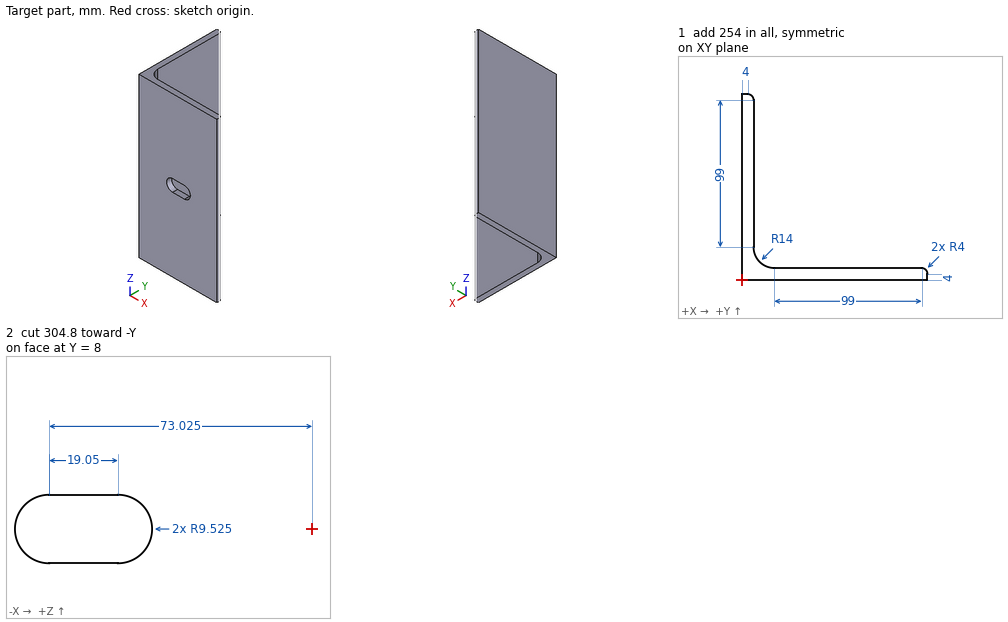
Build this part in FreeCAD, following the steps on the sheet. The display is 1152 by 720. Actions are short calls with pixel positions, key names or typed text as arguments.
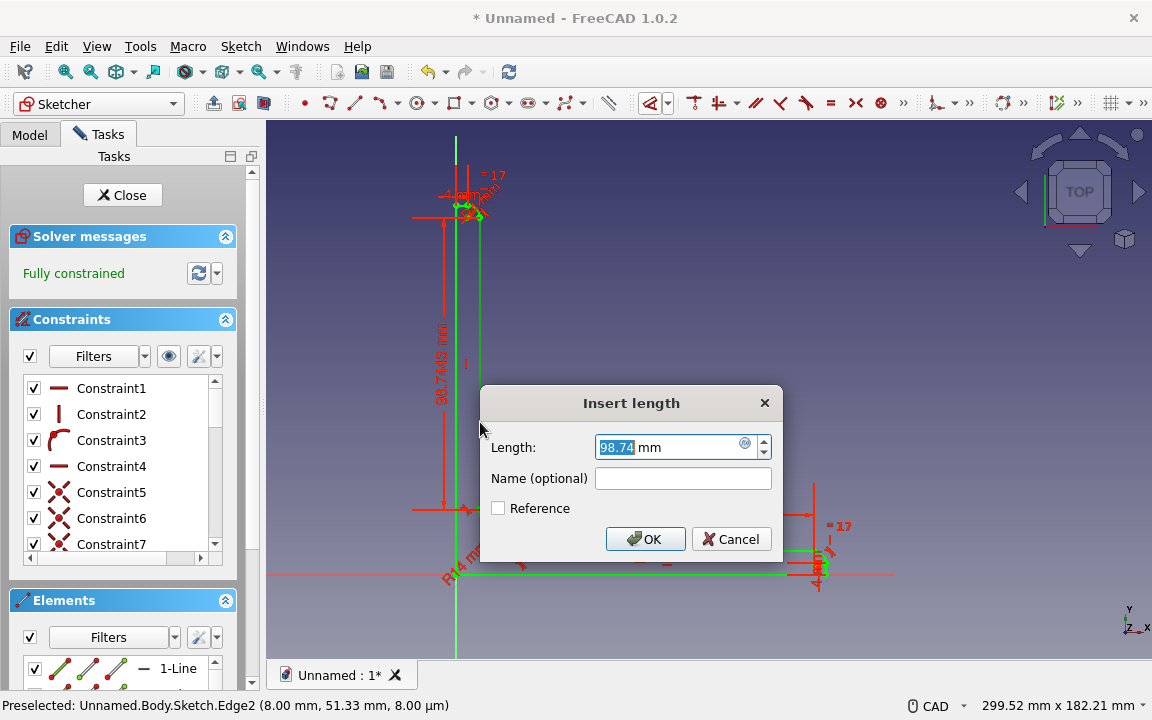
text(99)
key(Return)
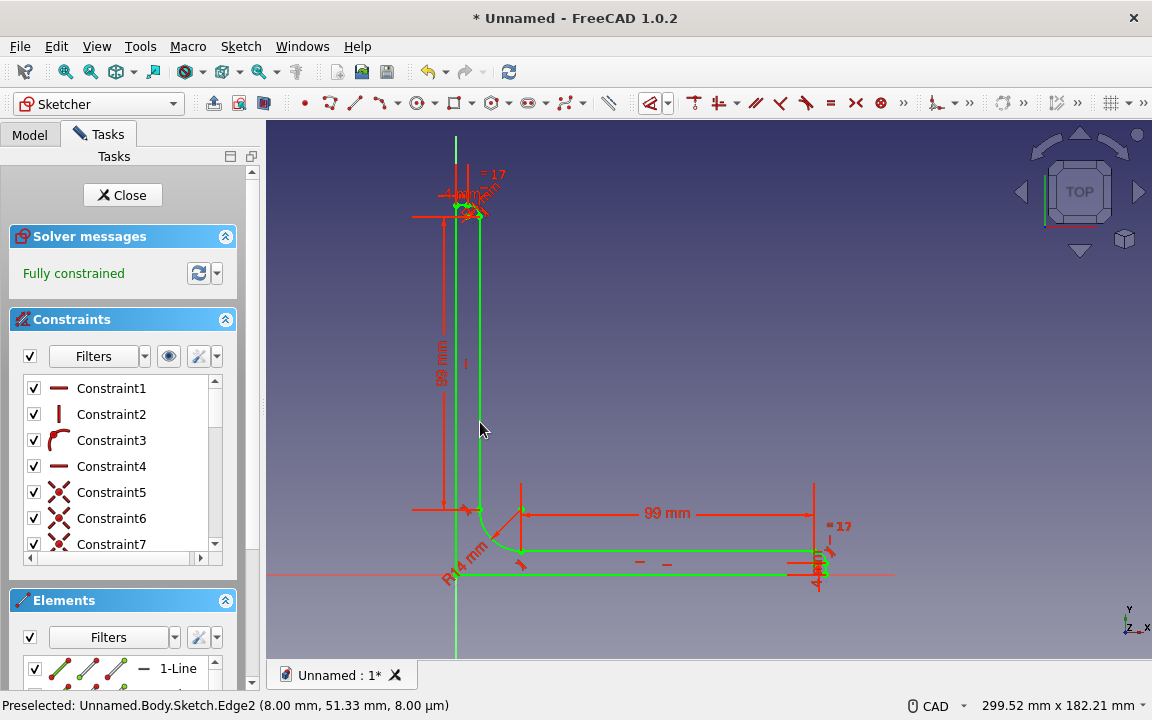
click(123, 195)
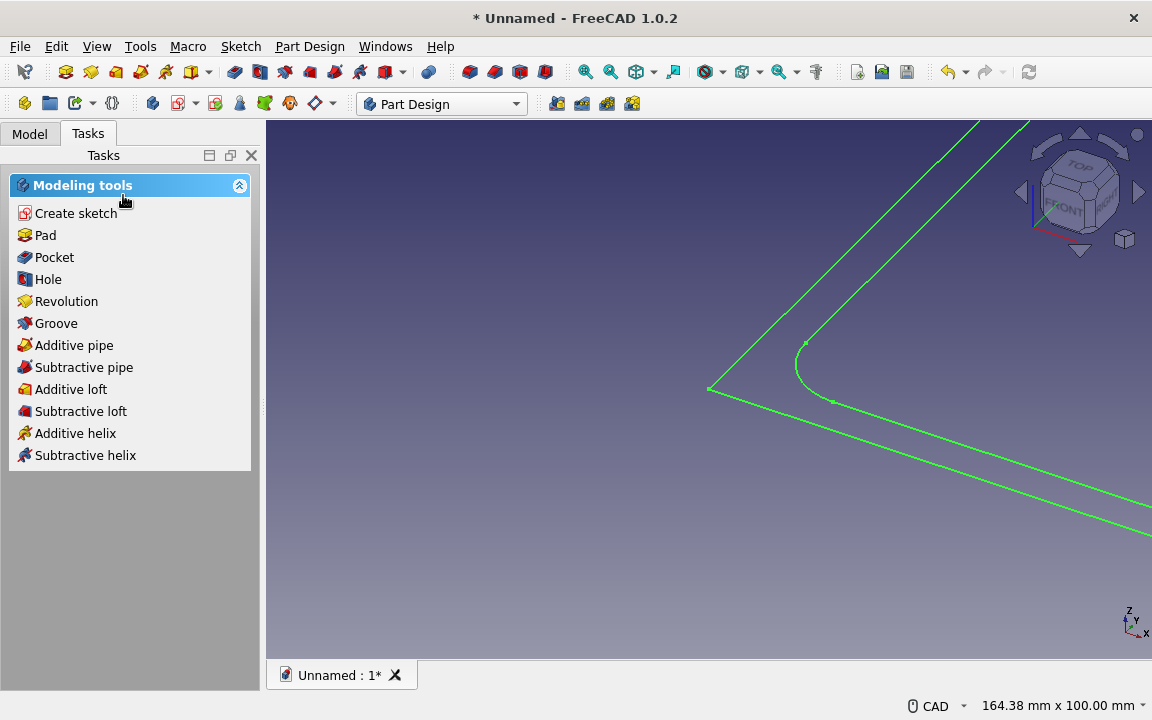
click(66, 72)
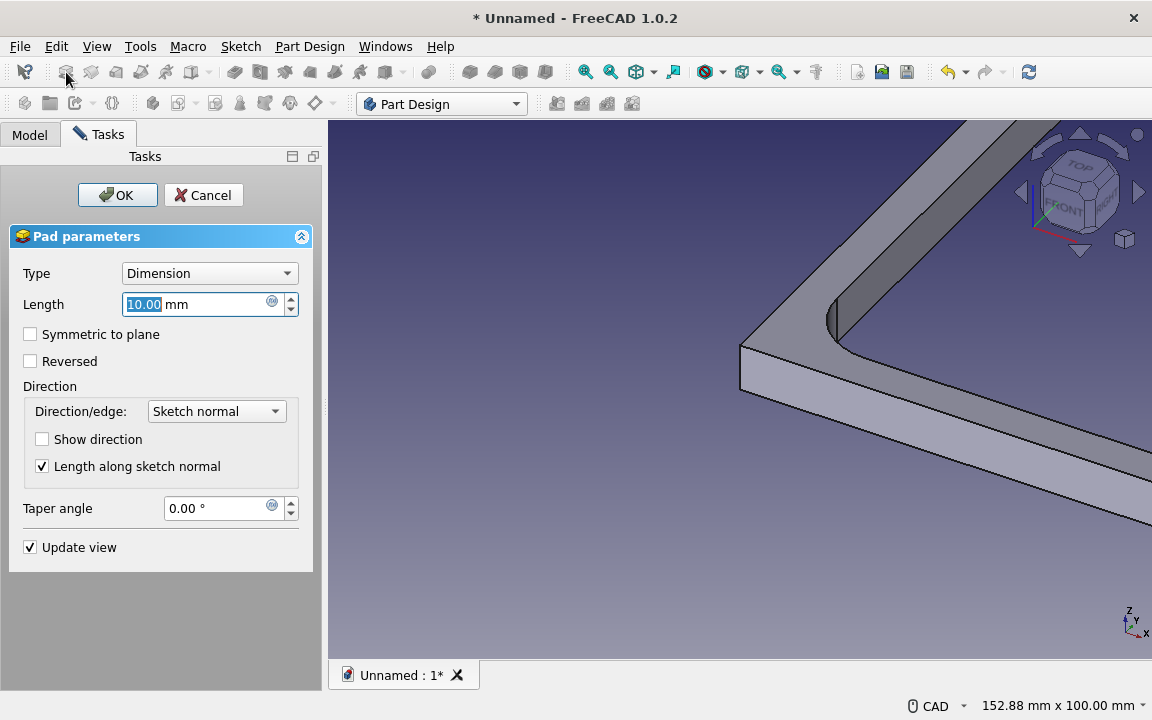
text(254)
key(Tab)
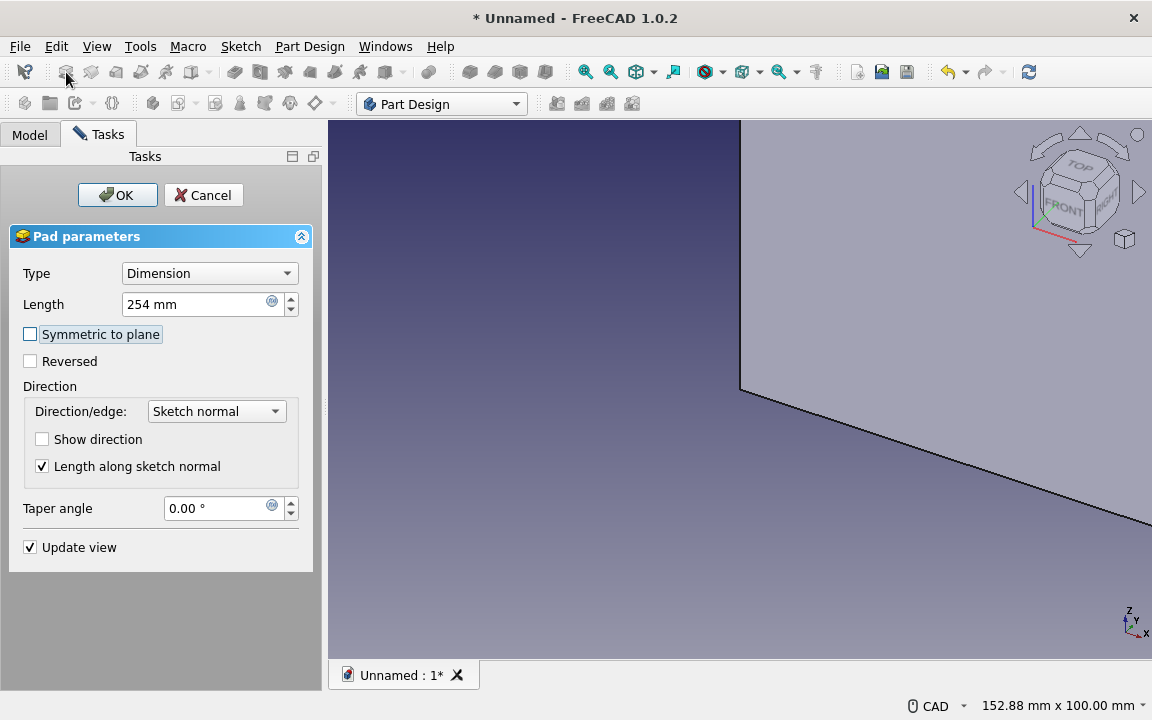
click(31, 334)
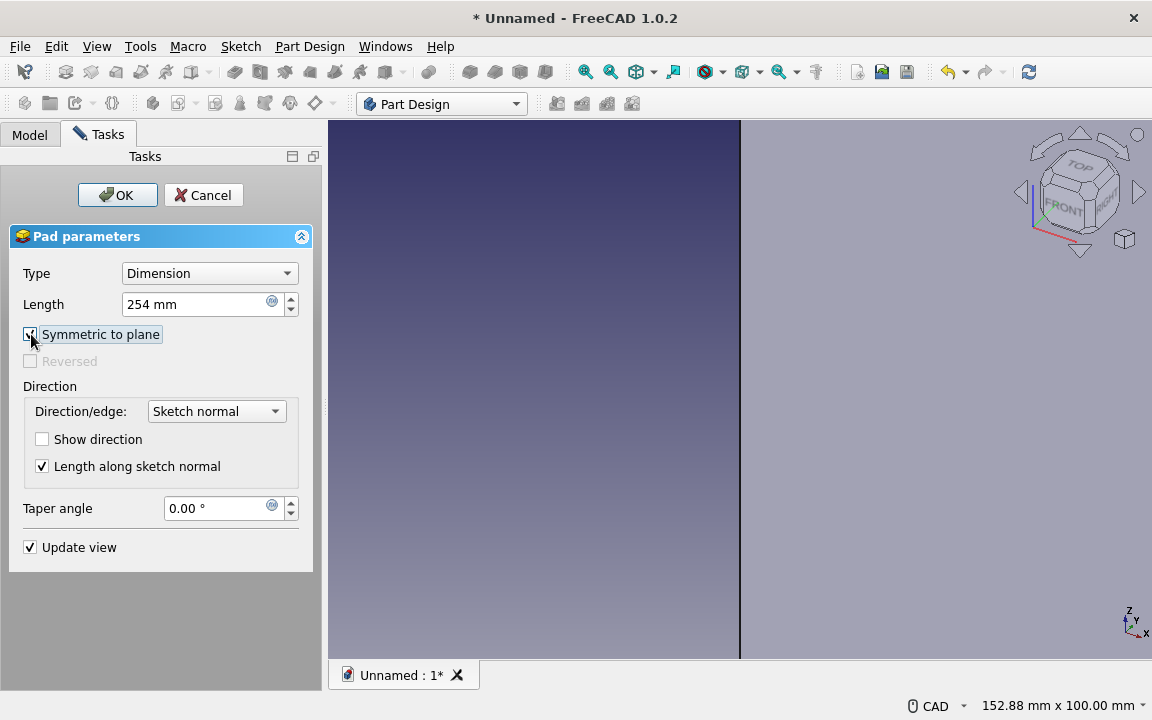
click(118, 195)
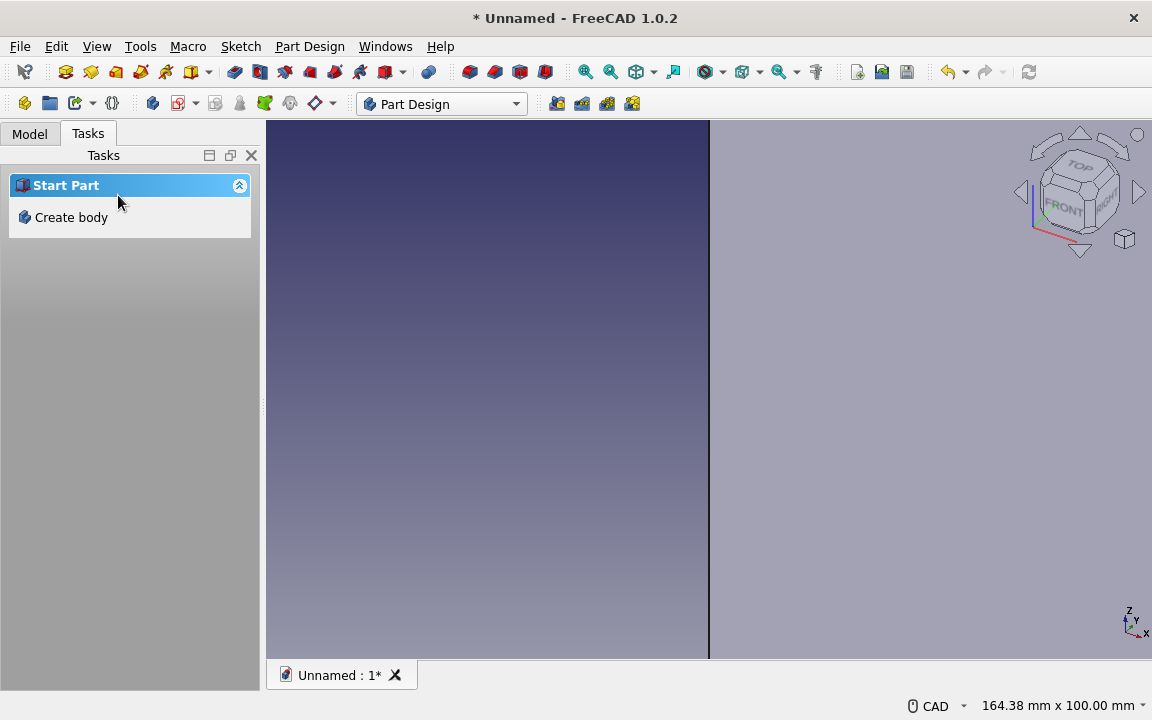
click(586, 72)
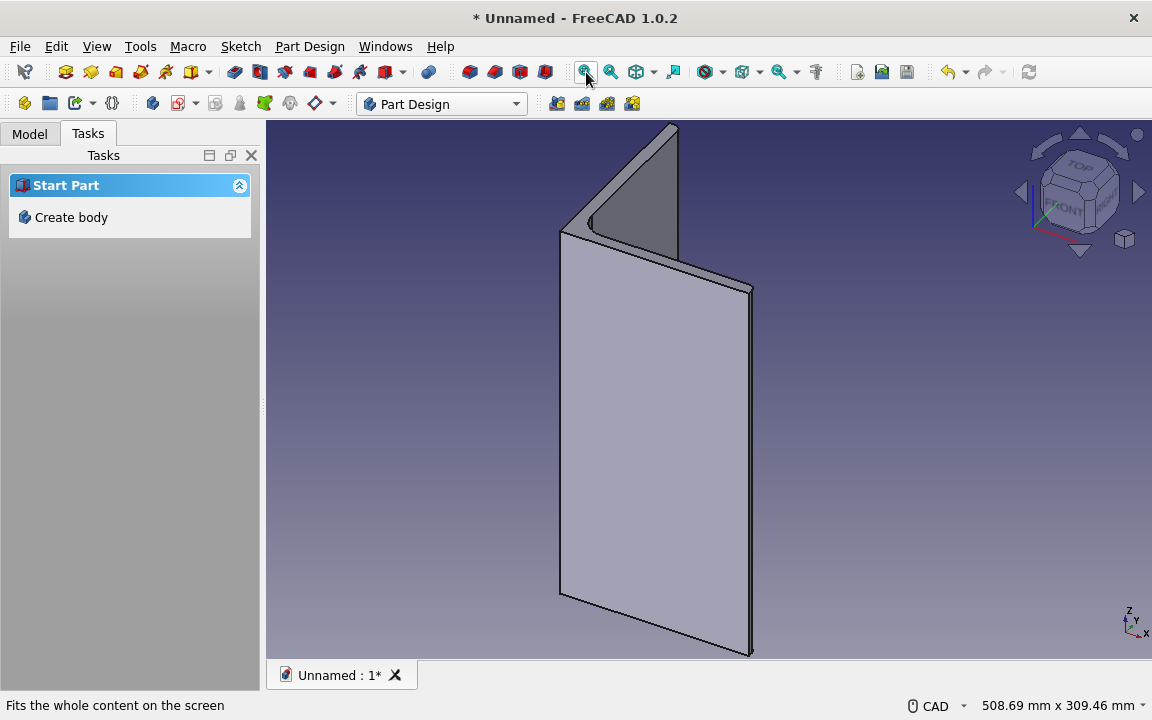
key(4)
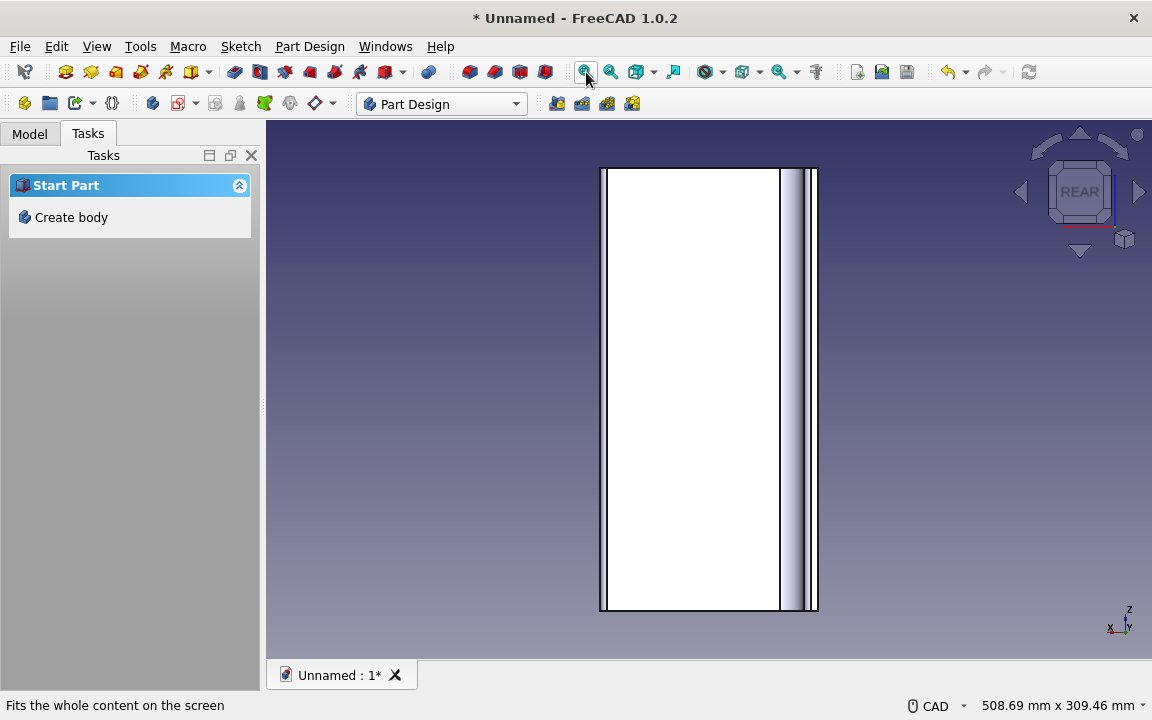
click(693, 262)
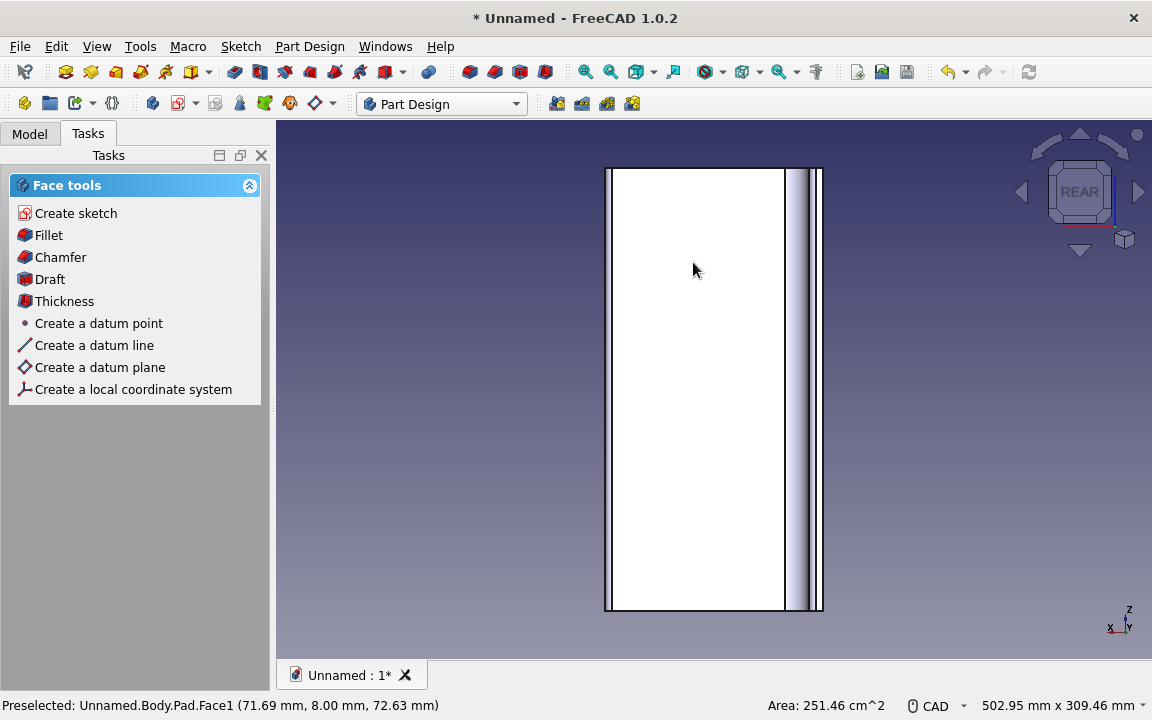
click(178, 104)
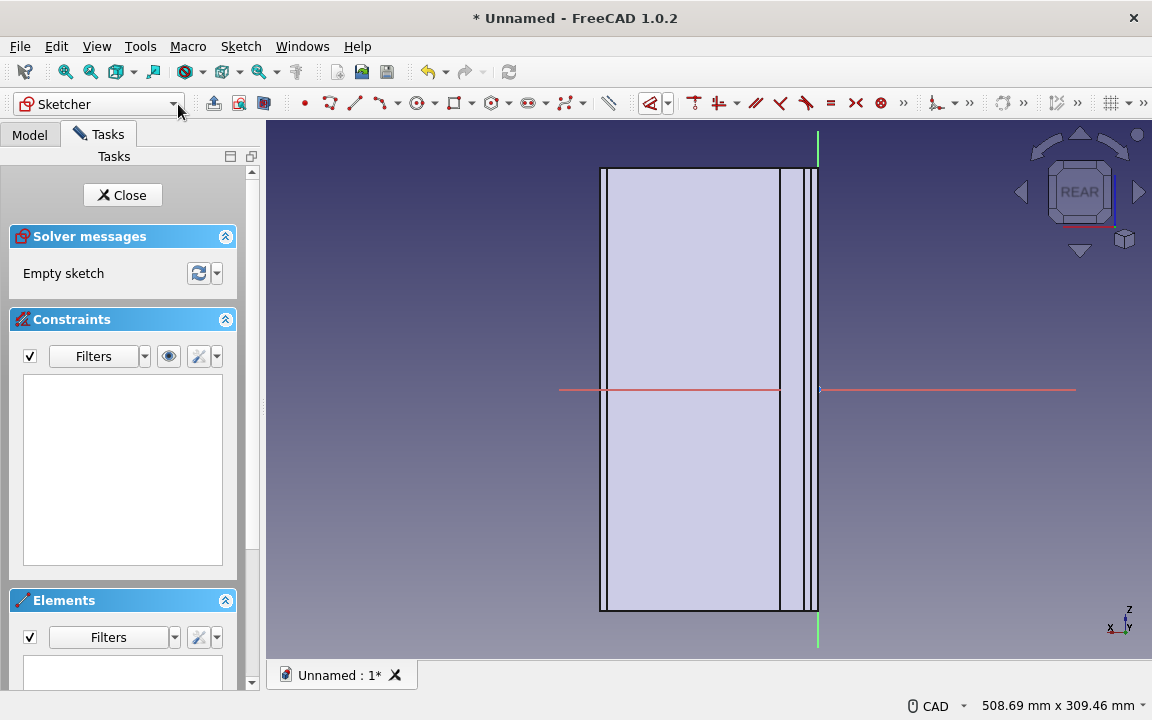
click(264, 104)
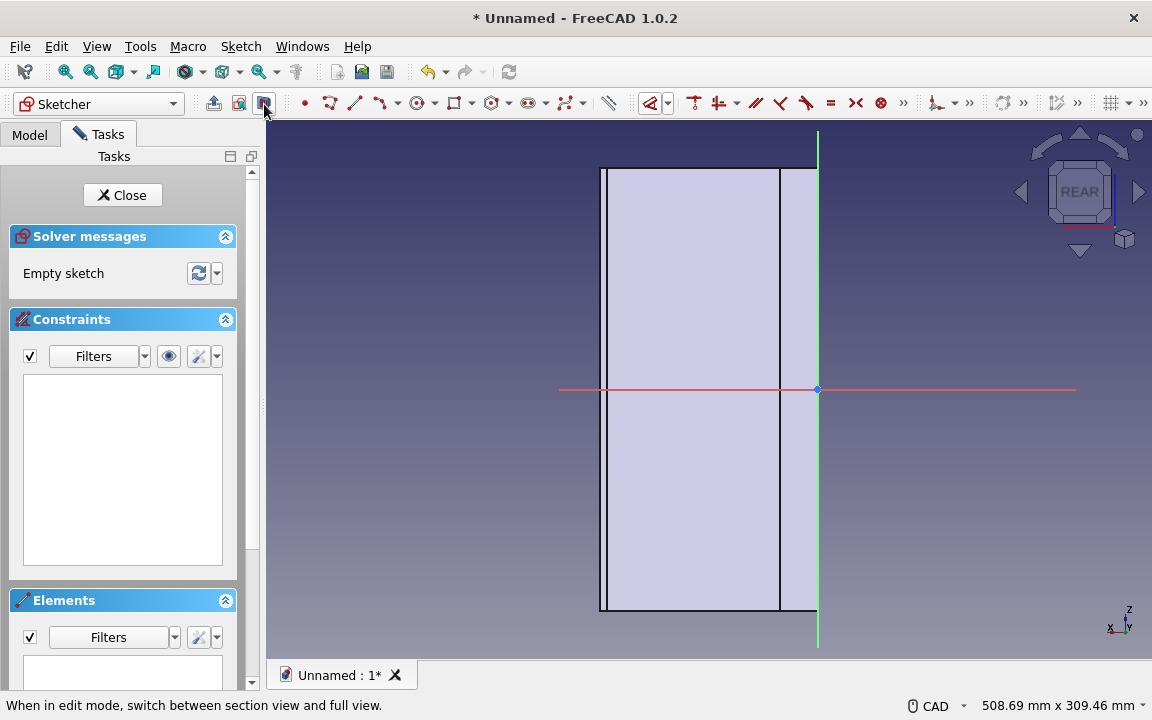
scroll(791, 389, up, 6)